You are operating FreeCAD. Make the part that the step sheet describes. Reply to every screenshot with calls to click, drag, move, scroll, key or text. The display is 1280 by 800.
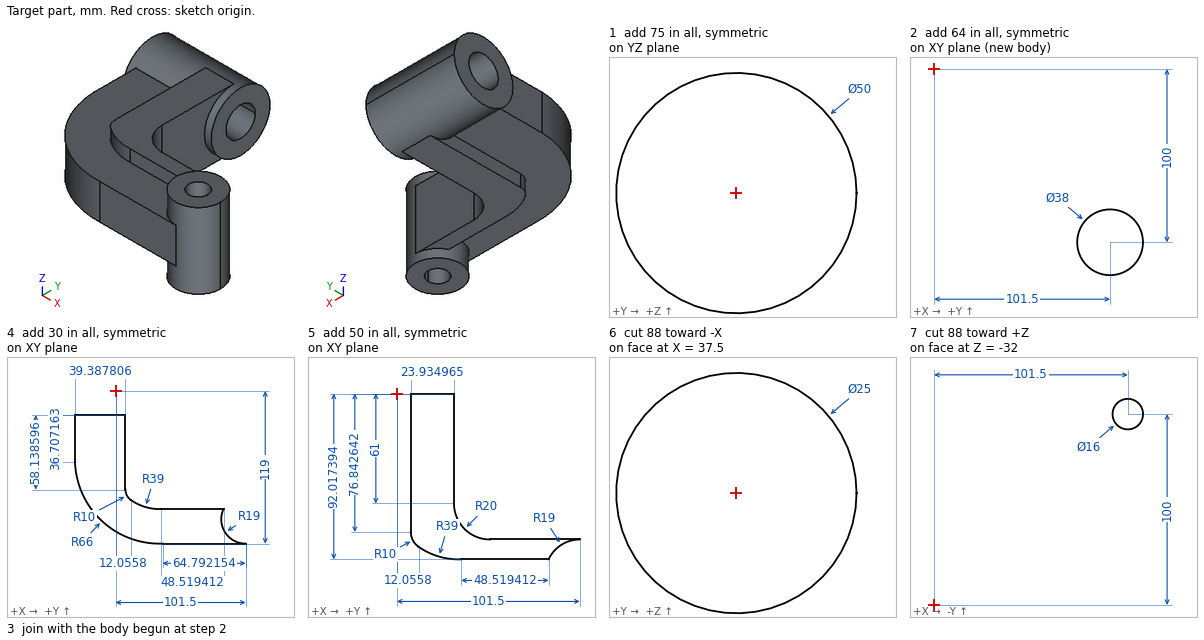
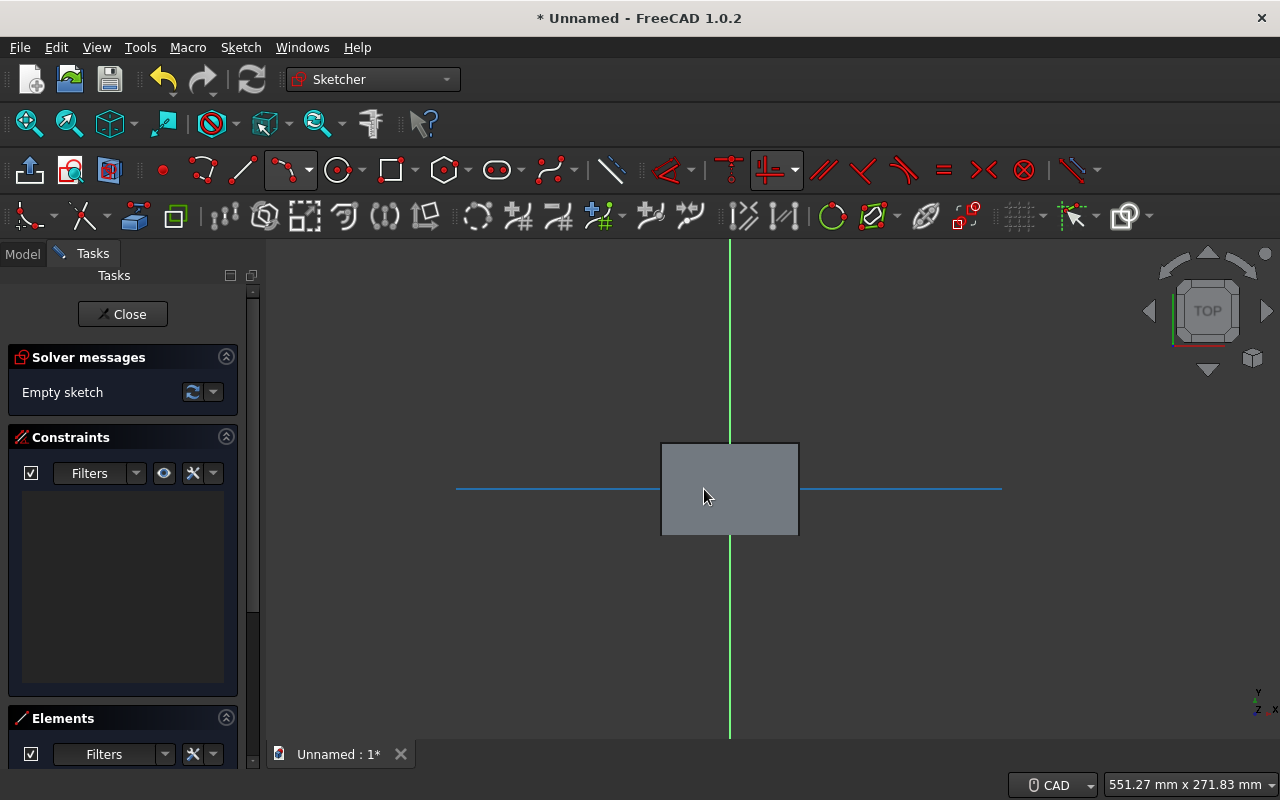
scroll(704, 489, down, 5)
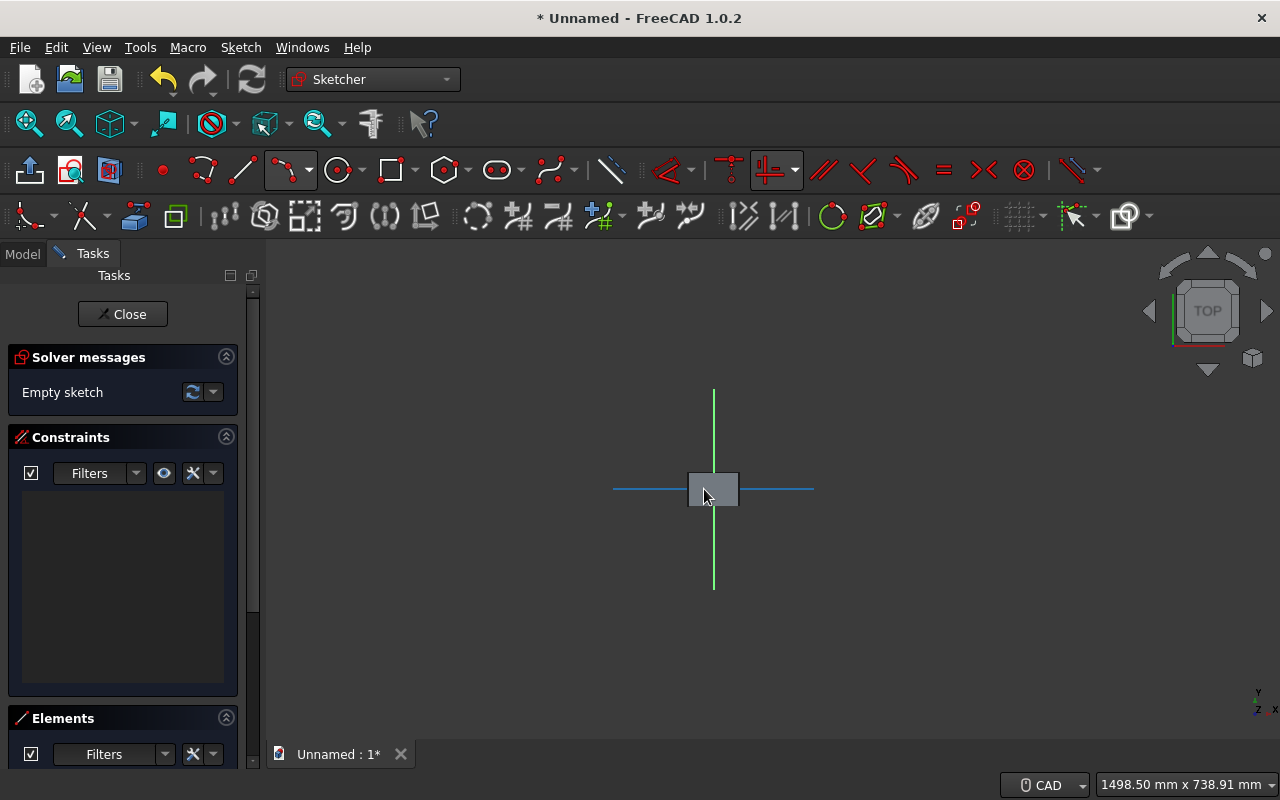
scroll(789, 563, up, 13)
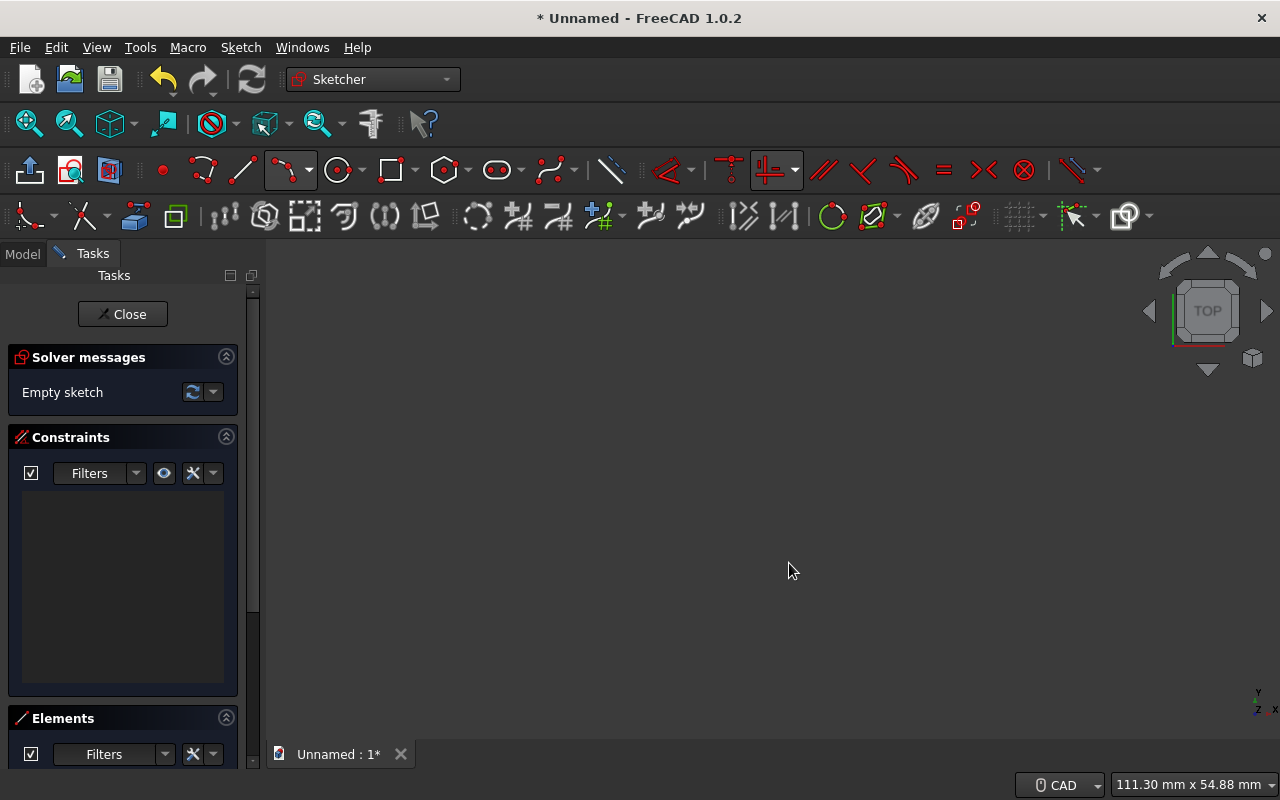
click(338, 170)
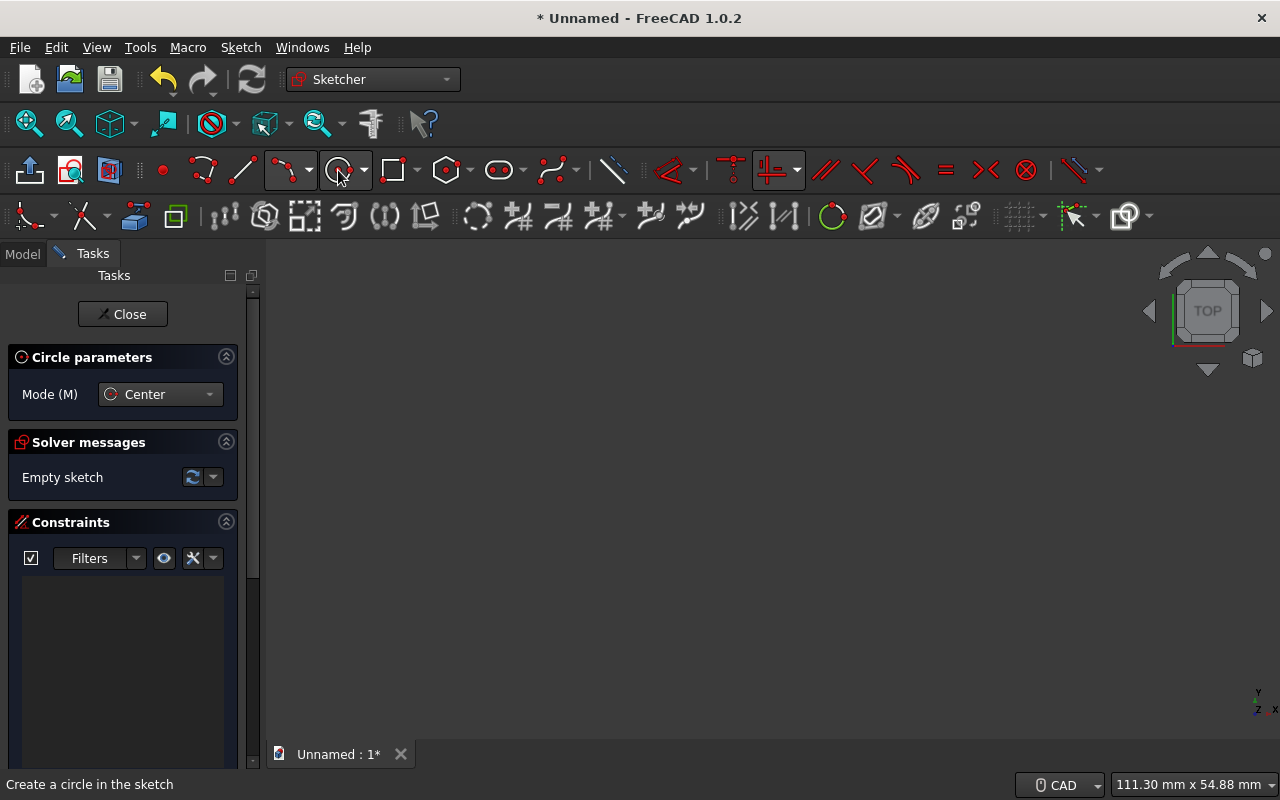
click(694, 475)
click(816, 353)
key(Escape)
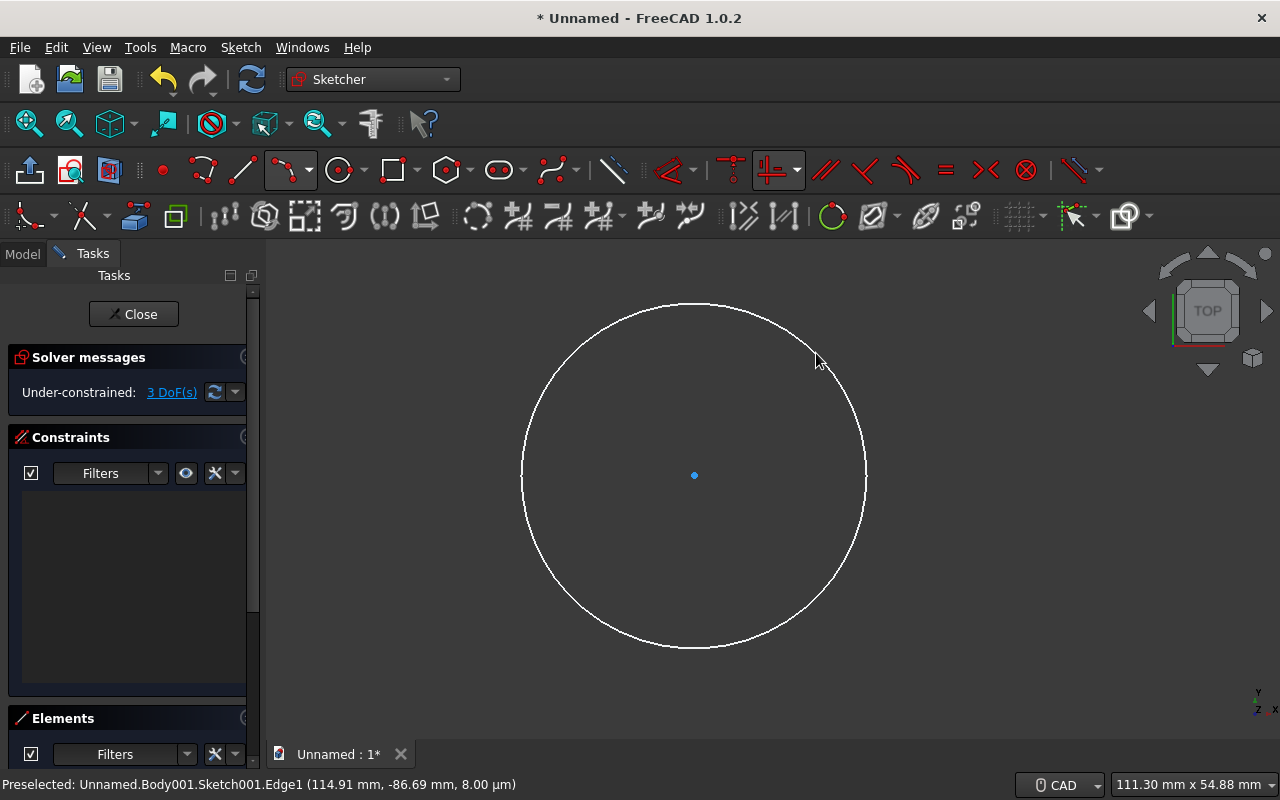
click(668, 170)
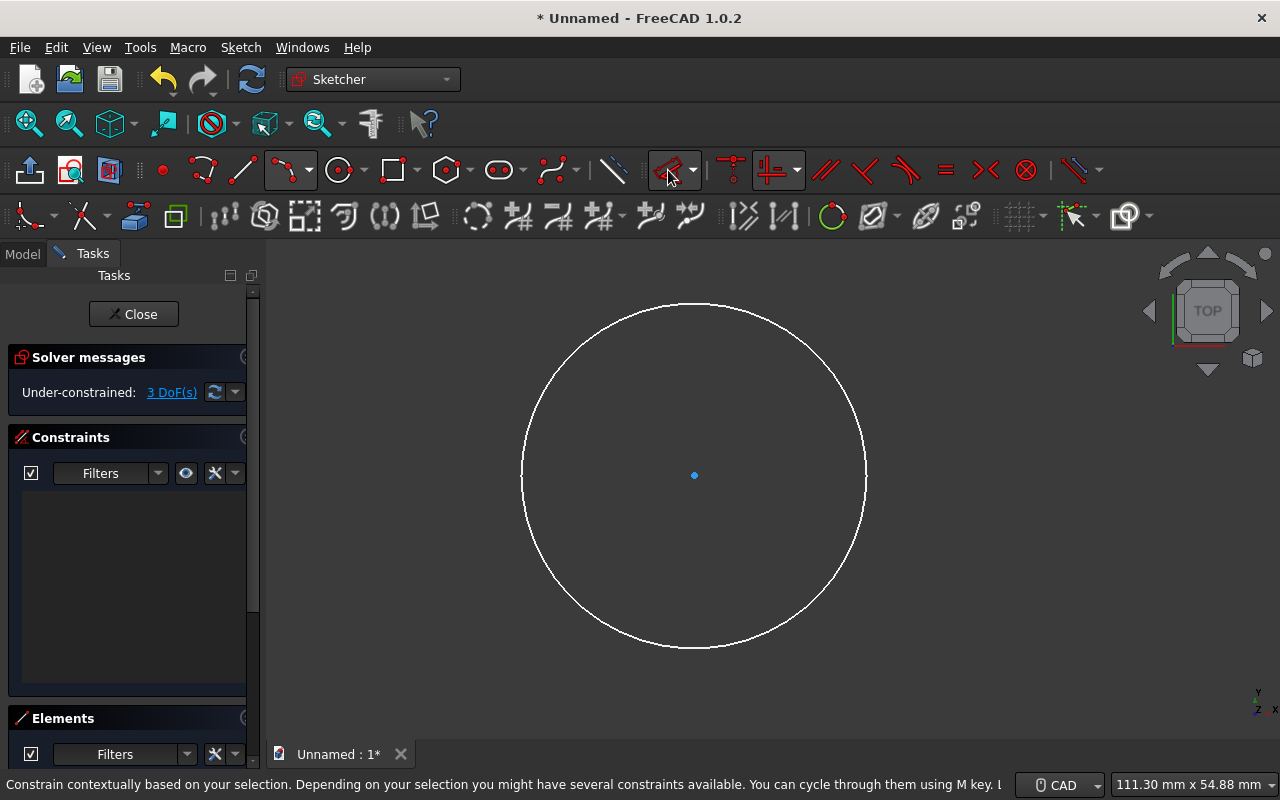
click(816, 354)
click(839, 331)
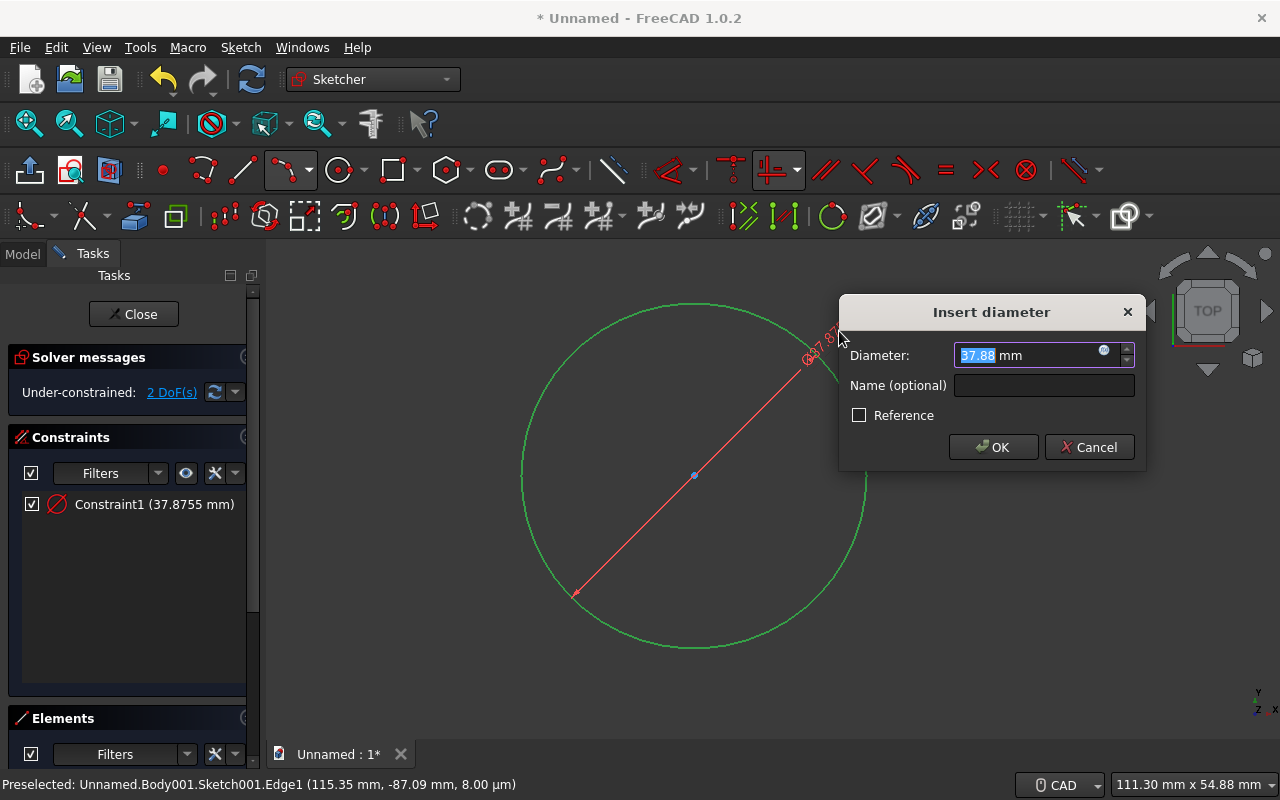
text(38)
key(Return)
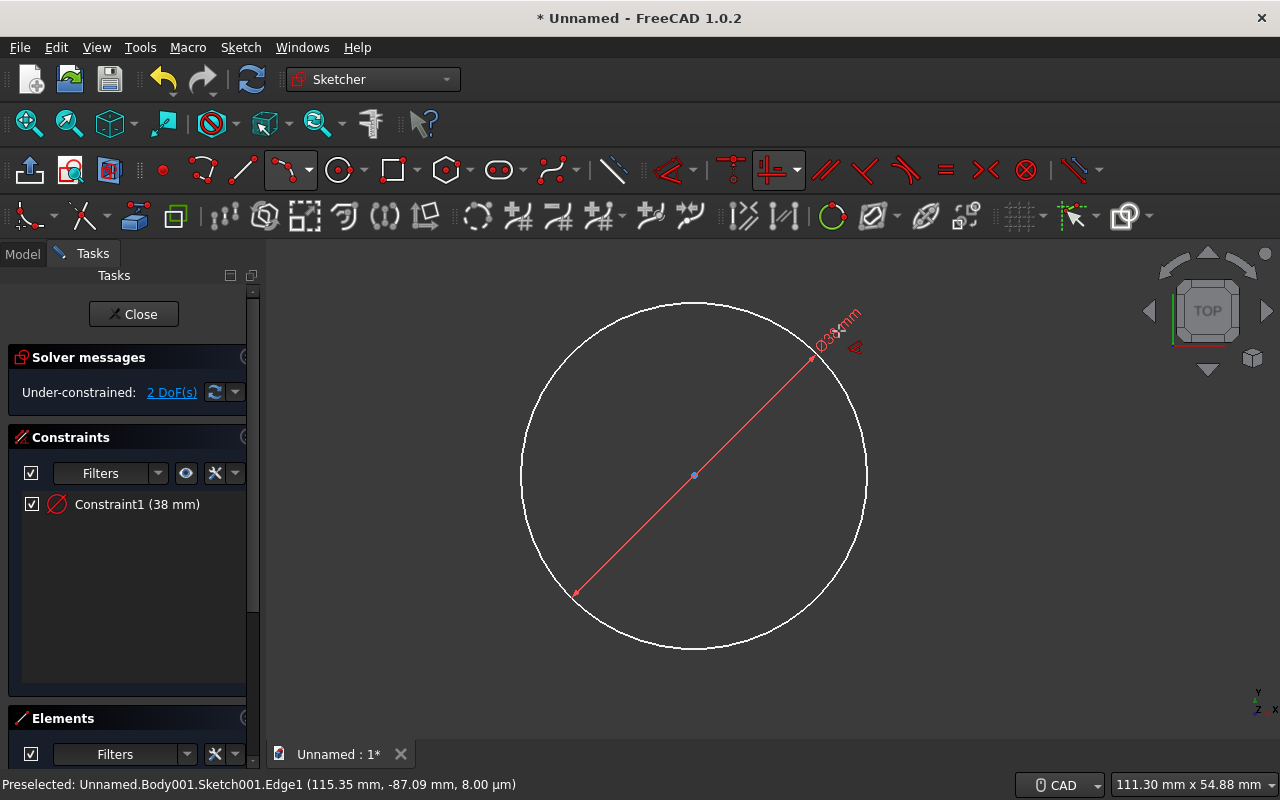
click(694, 476)
click(728, 371)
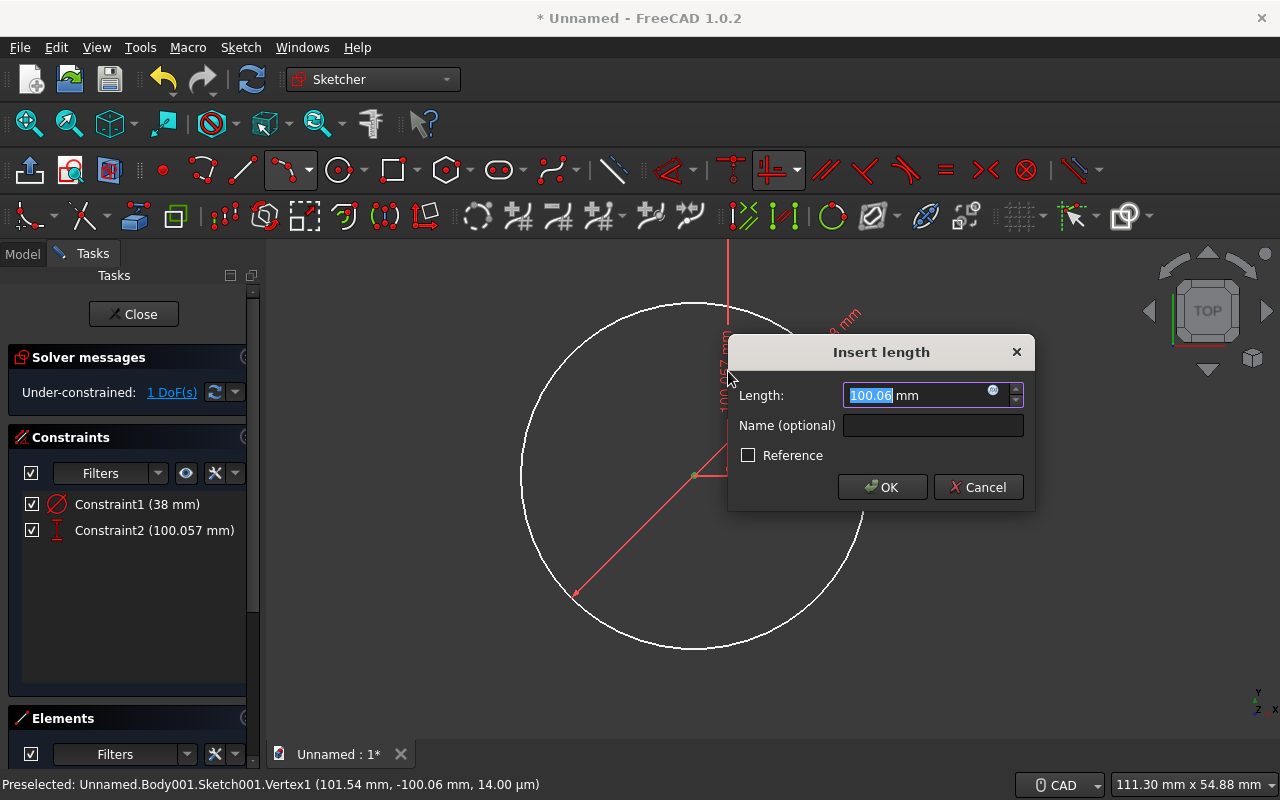
text(100)
key(Return)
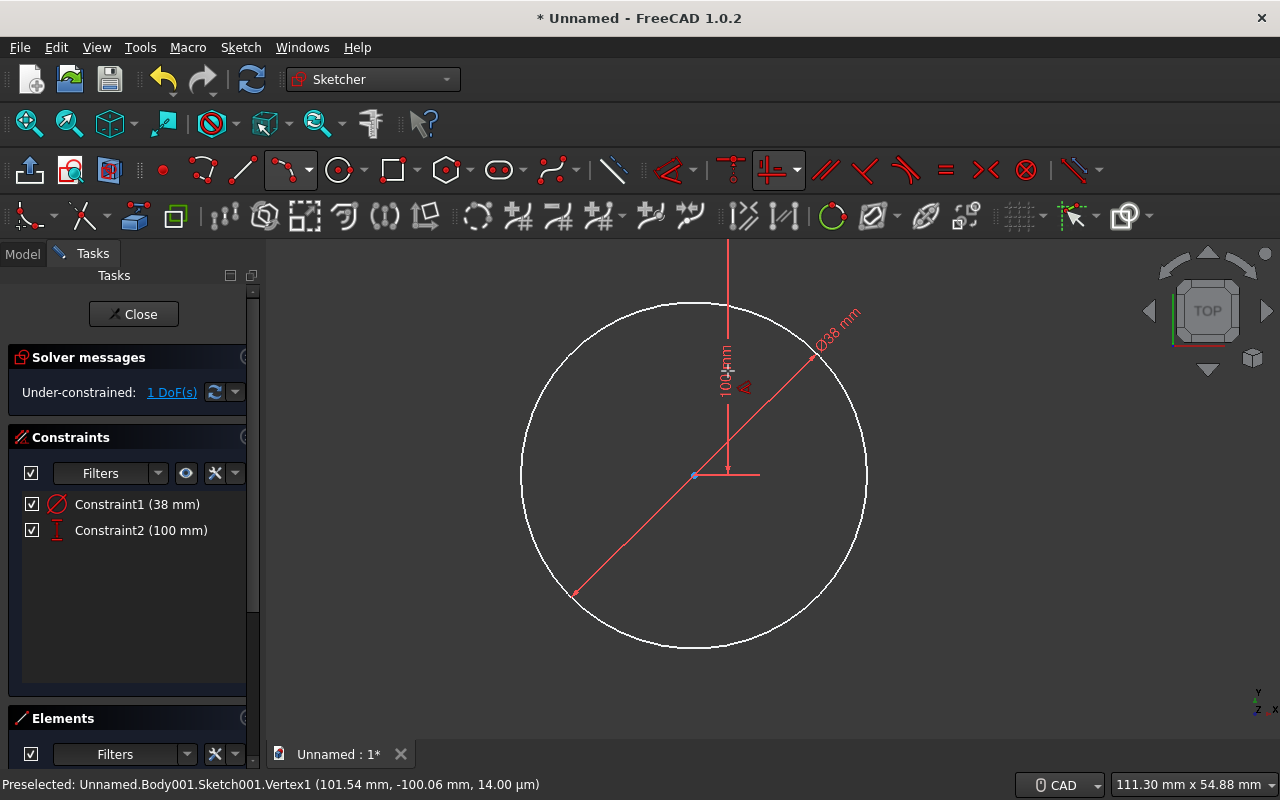
click(694, 475)
click(494, 509)